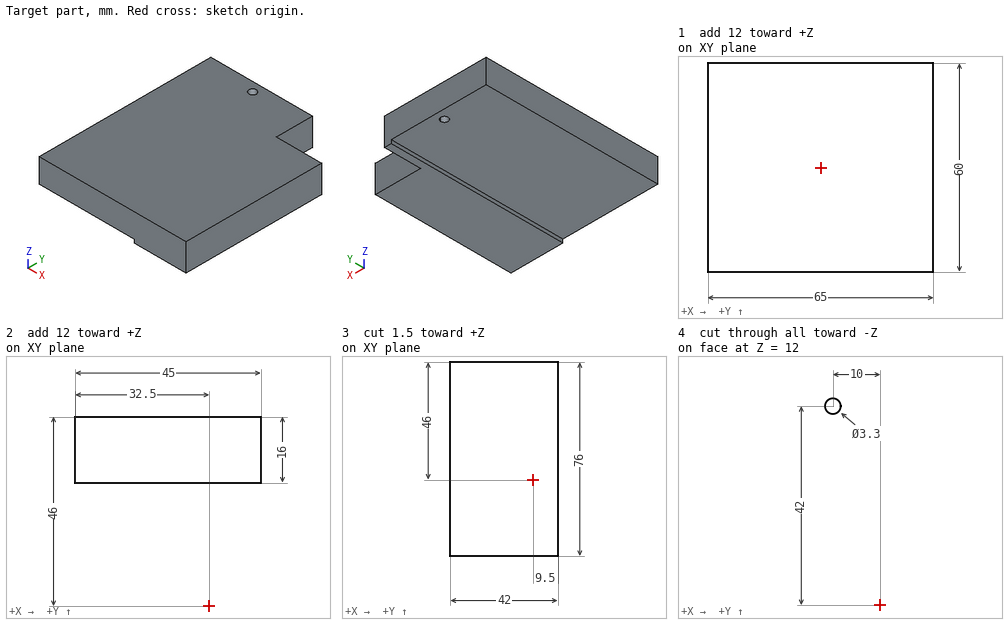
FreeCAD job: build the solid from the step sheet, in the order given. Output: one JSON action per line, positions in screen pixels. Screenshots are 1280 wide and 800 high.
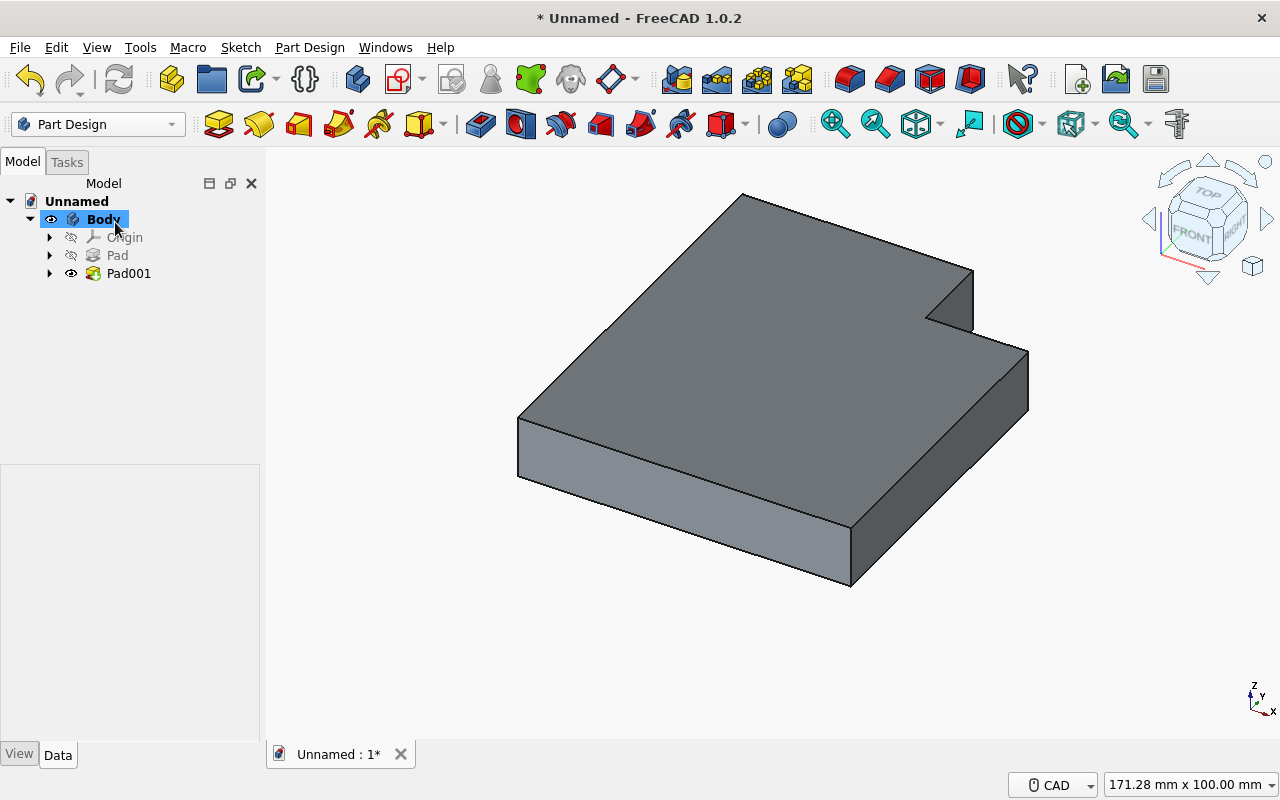
{"action": "left_click", "coordinate": [398, 80]}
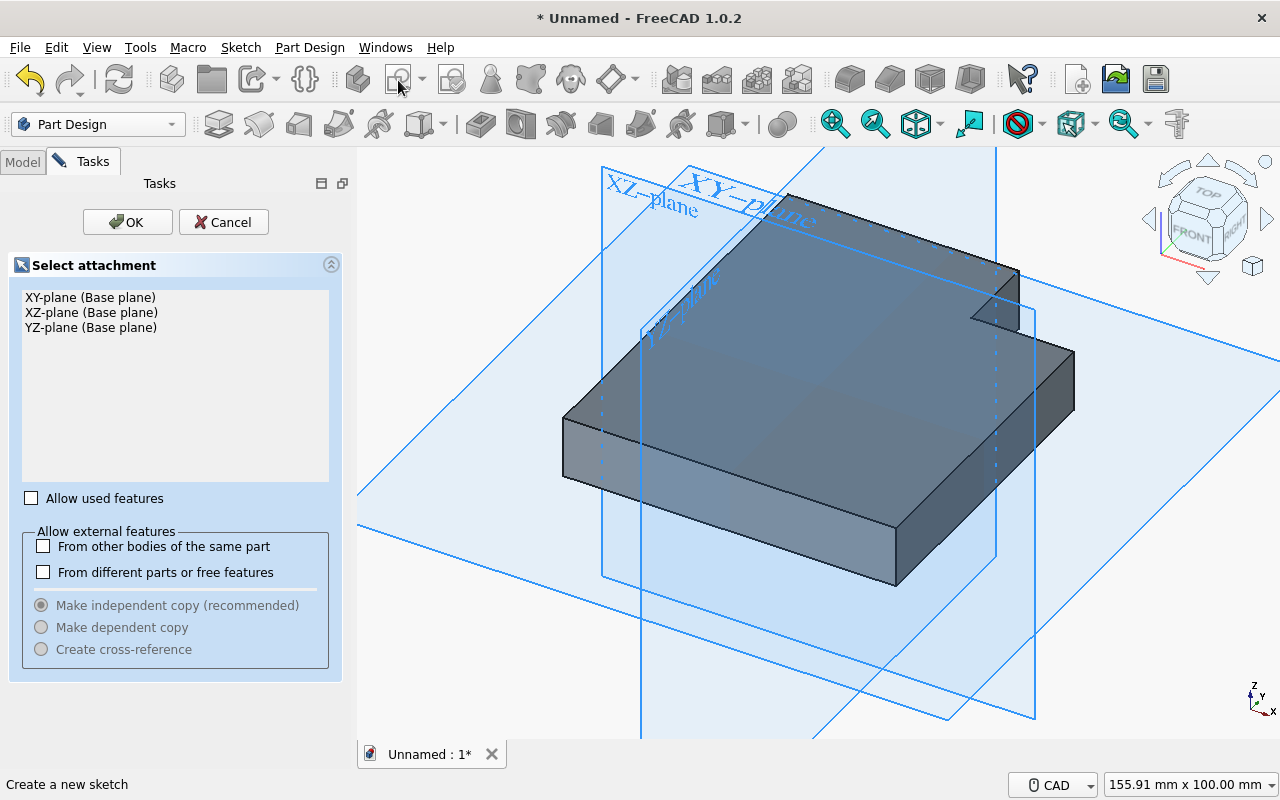
{"action": "left_click", "coordinate": [82, 298]}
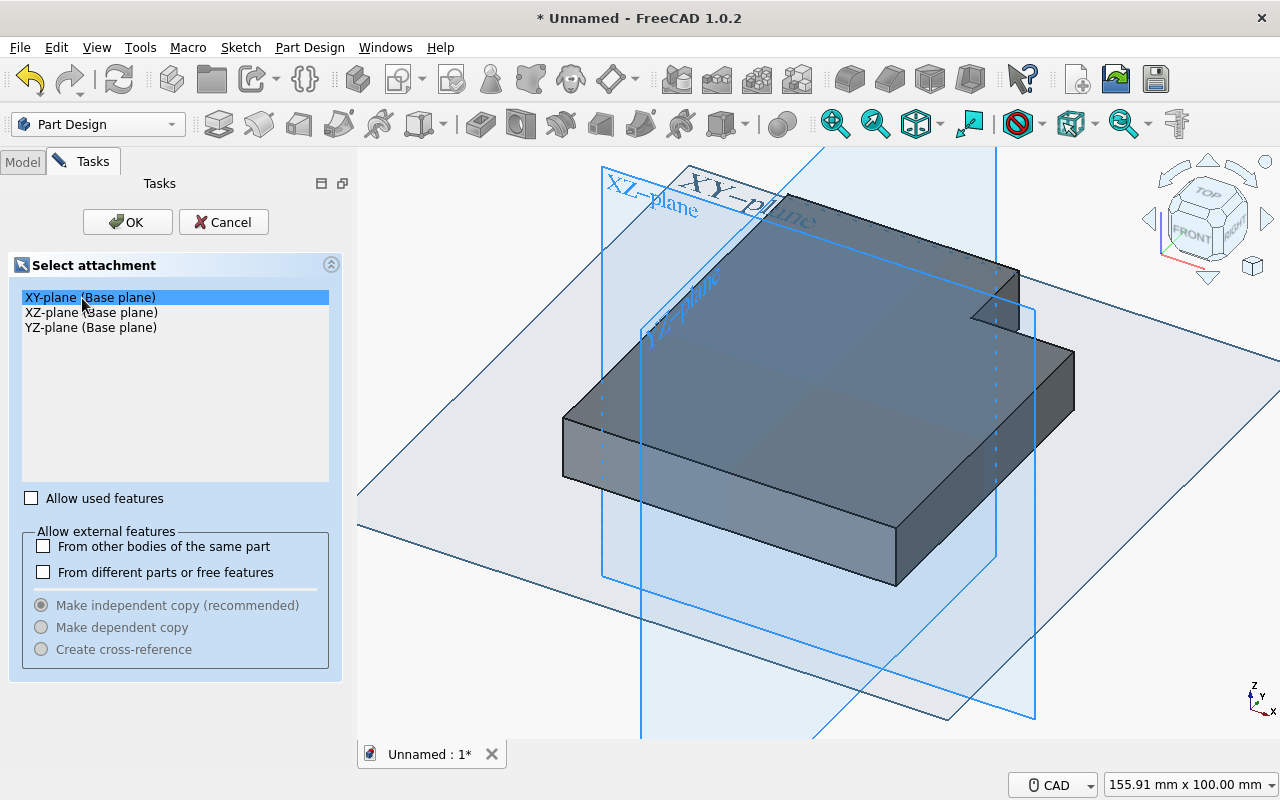
{"action": "left_click", "coordinate": [128, 222]}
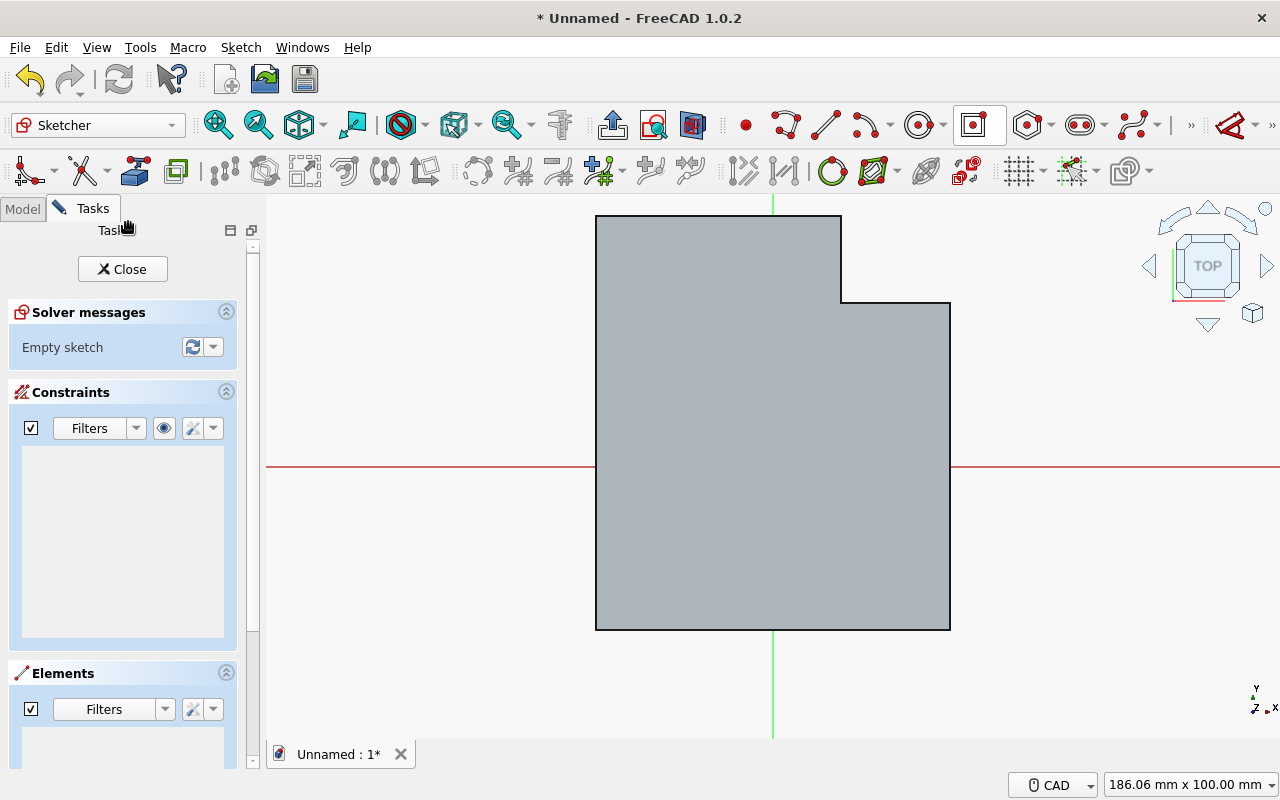
{"action": "left_click", "coordinate": [694, 126]}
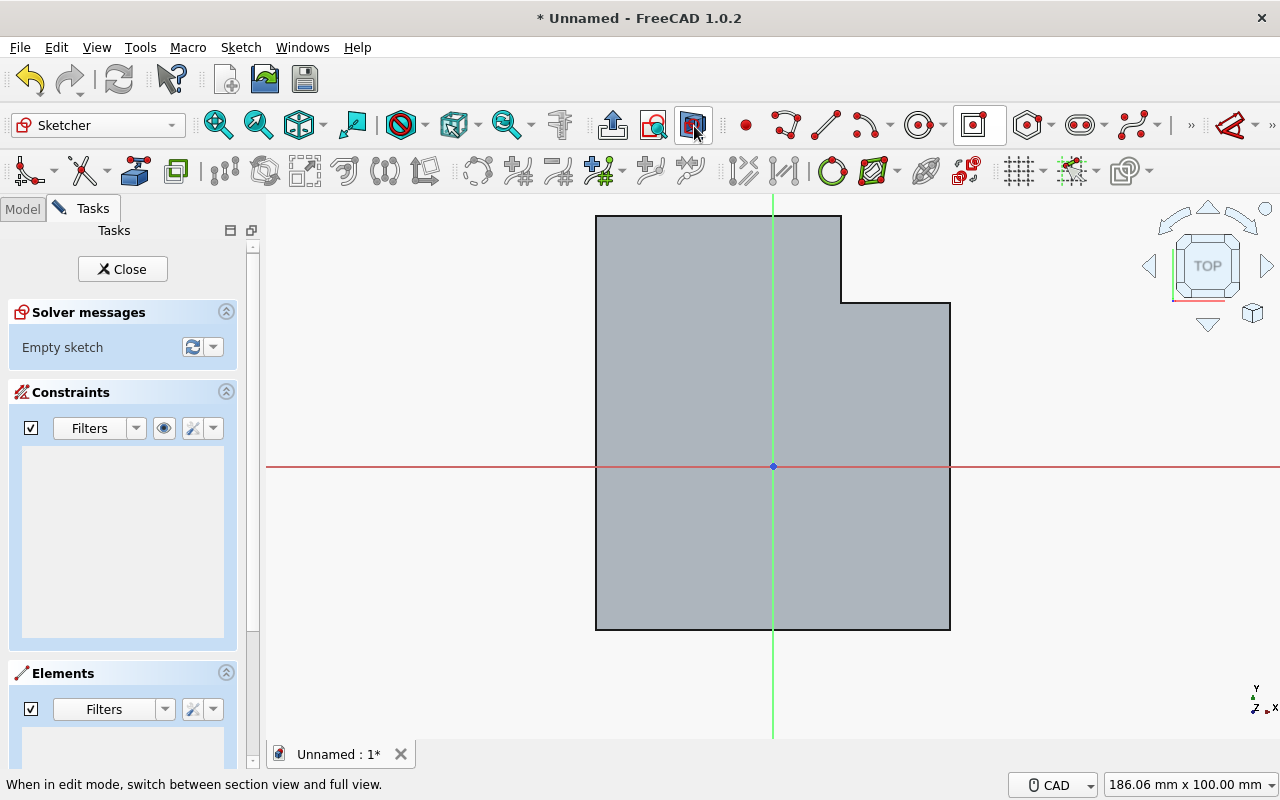
{"action": "scroll", "coordinate": [678, 663], "scroll_direction": "down", "scroll_amount": 1}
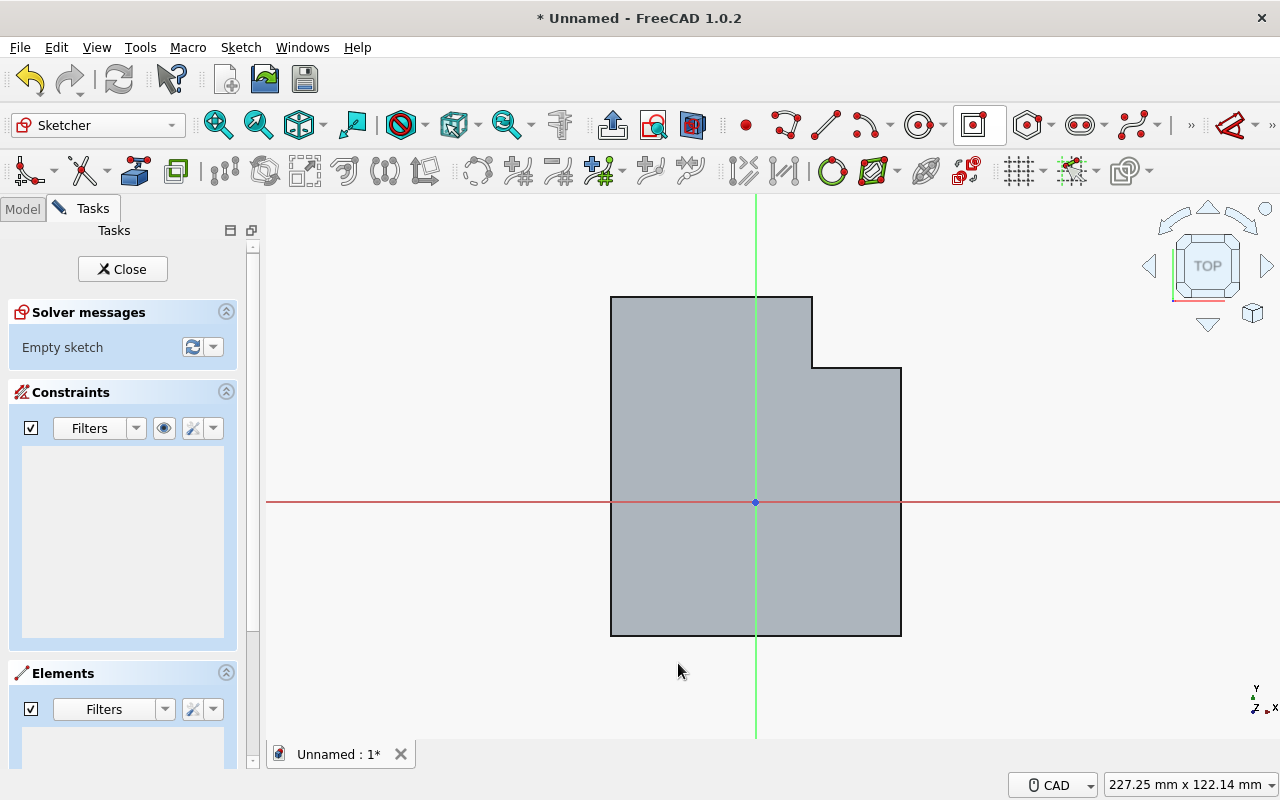
{"action": "key", "text": "g r"}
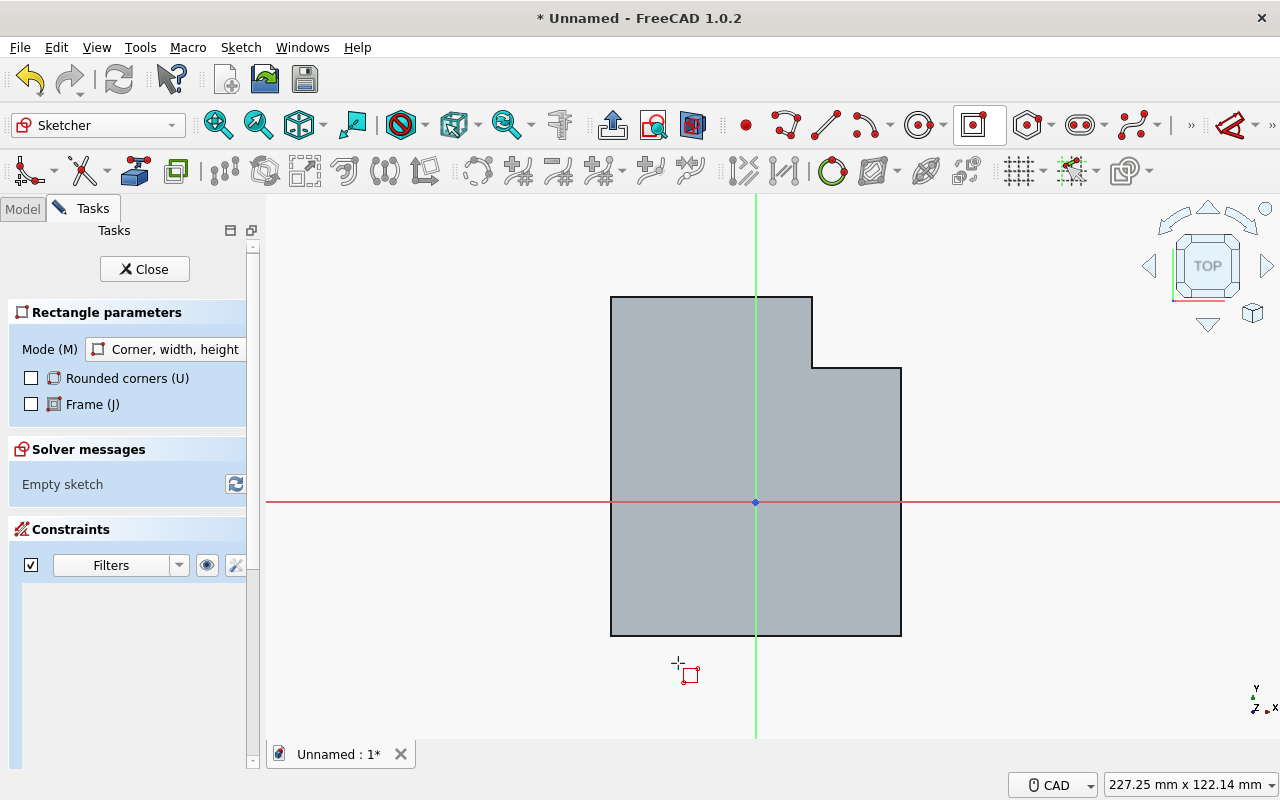
{"action": "left_click", "coordinate": [611, 297]}
{"action": "mouse_move", "coordinate": [798, 636]}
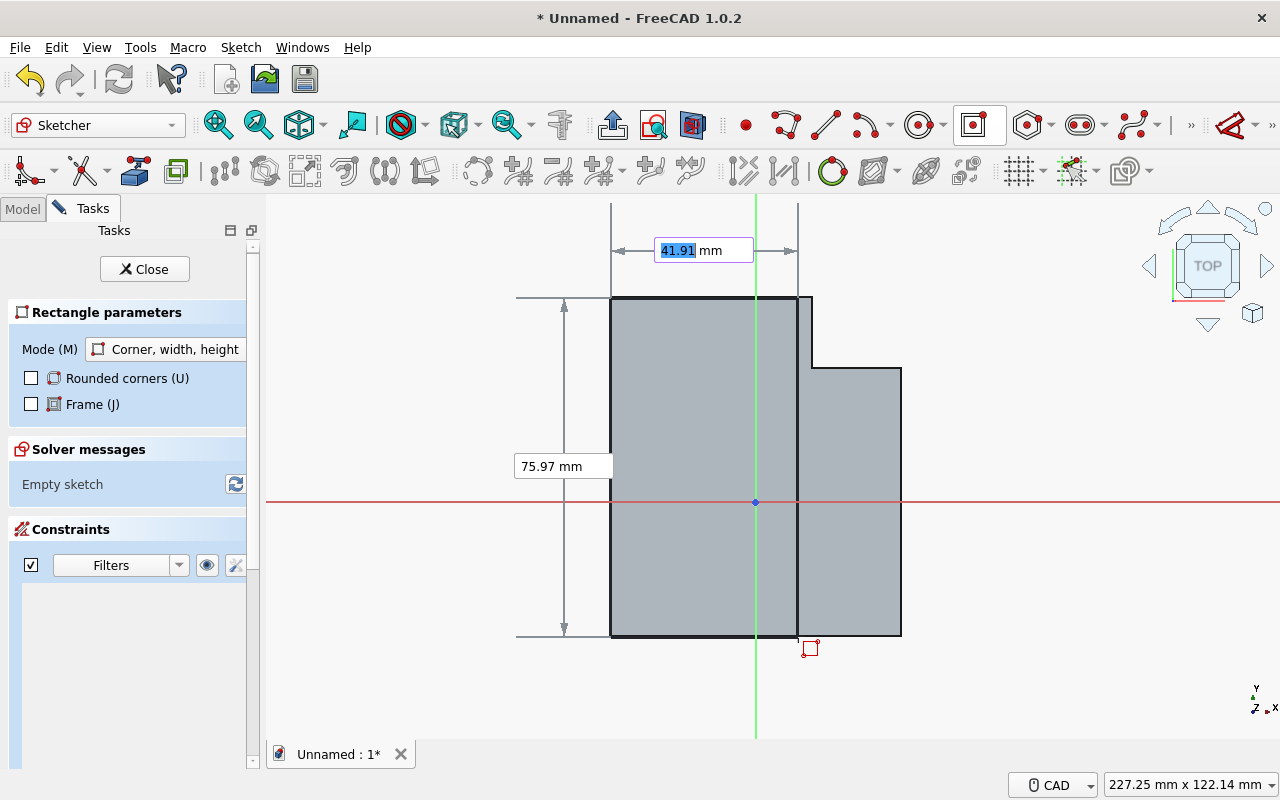
{"action": "type", "text": "42"}
{"action": "key", "text": "Tab"}
{"action": "type", "text": "76"}
{"action": "key", "text": "Return"}
{"action": "key", "text": "Escape"}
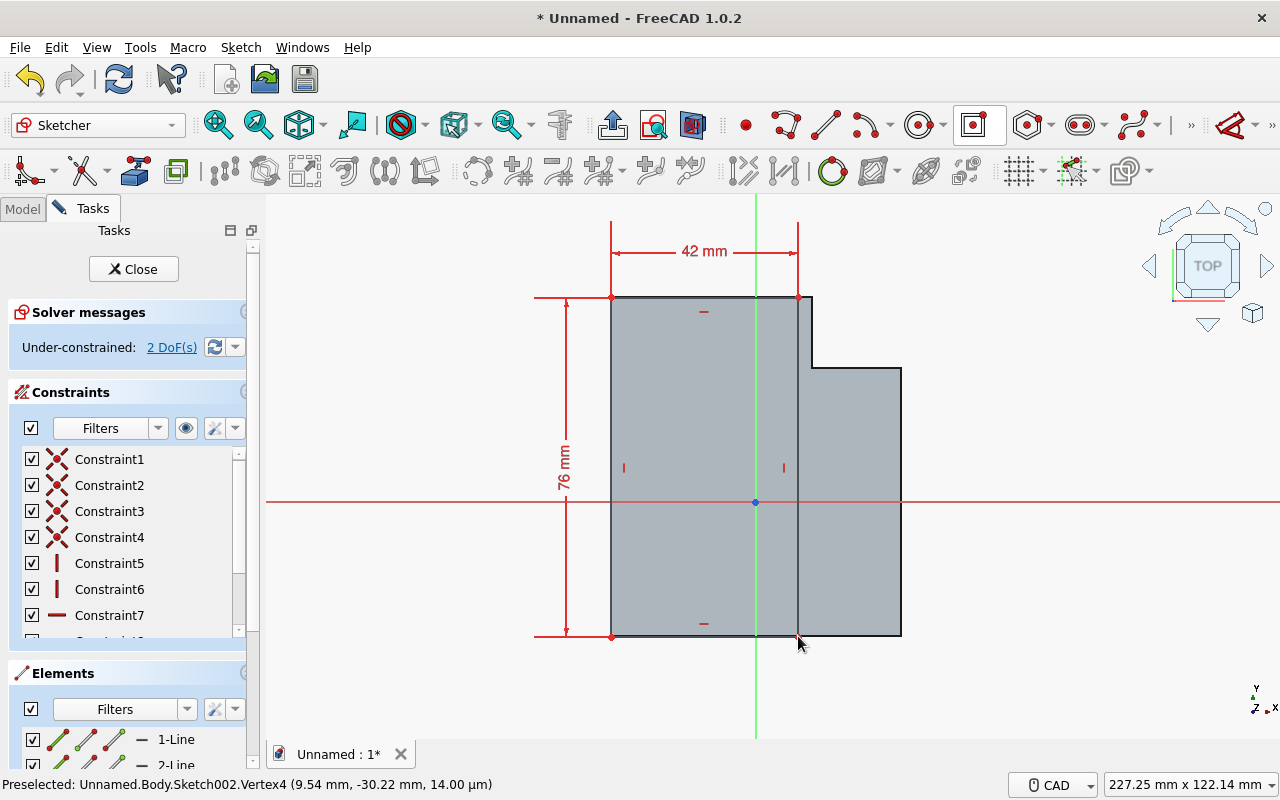
{"action": "left_click", "coordinate": [1230, 126]}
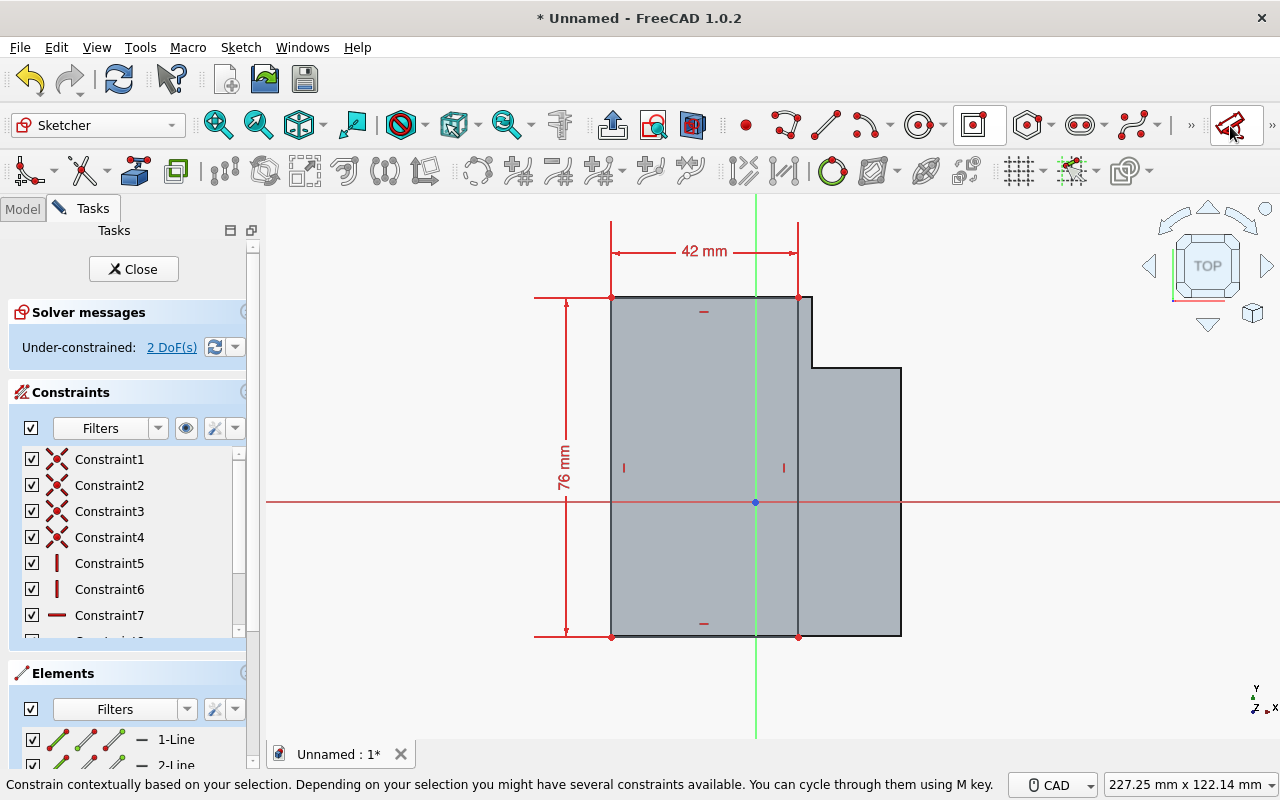
{"action": "left_click", "coordinate": [611, 298]}
{"action": "left_click", "coordinate": [577, 400]}